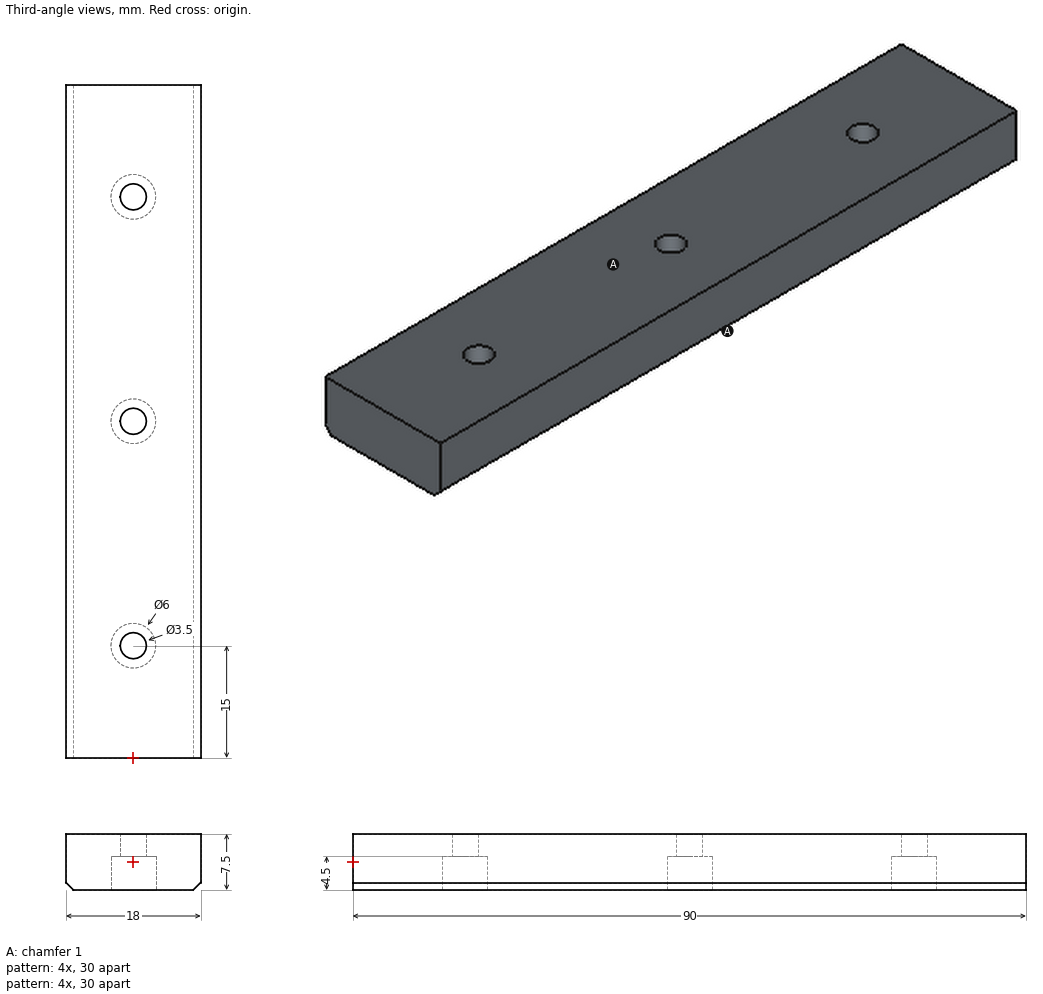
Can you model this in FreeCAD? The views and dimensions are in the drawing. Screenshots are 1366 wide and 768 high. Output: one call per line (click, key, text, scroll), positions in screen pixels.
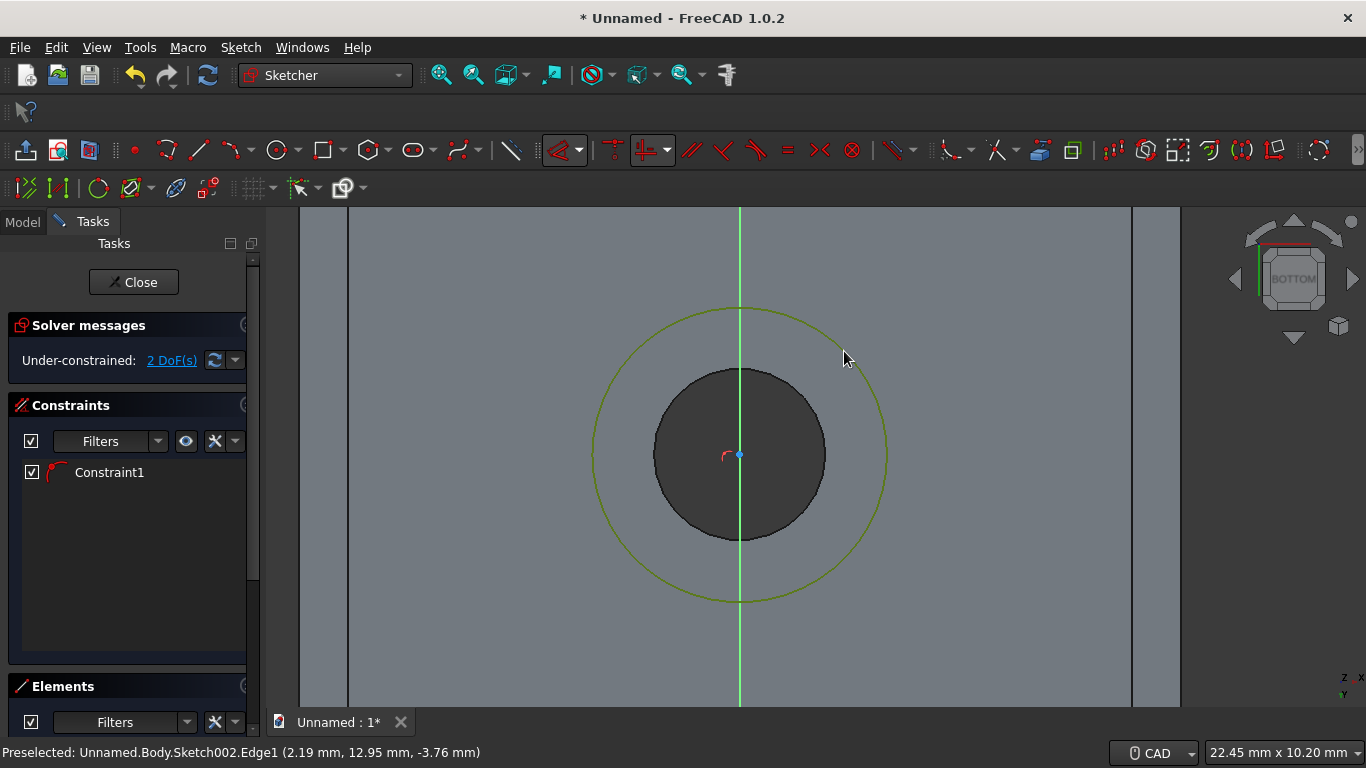
click(582, 150)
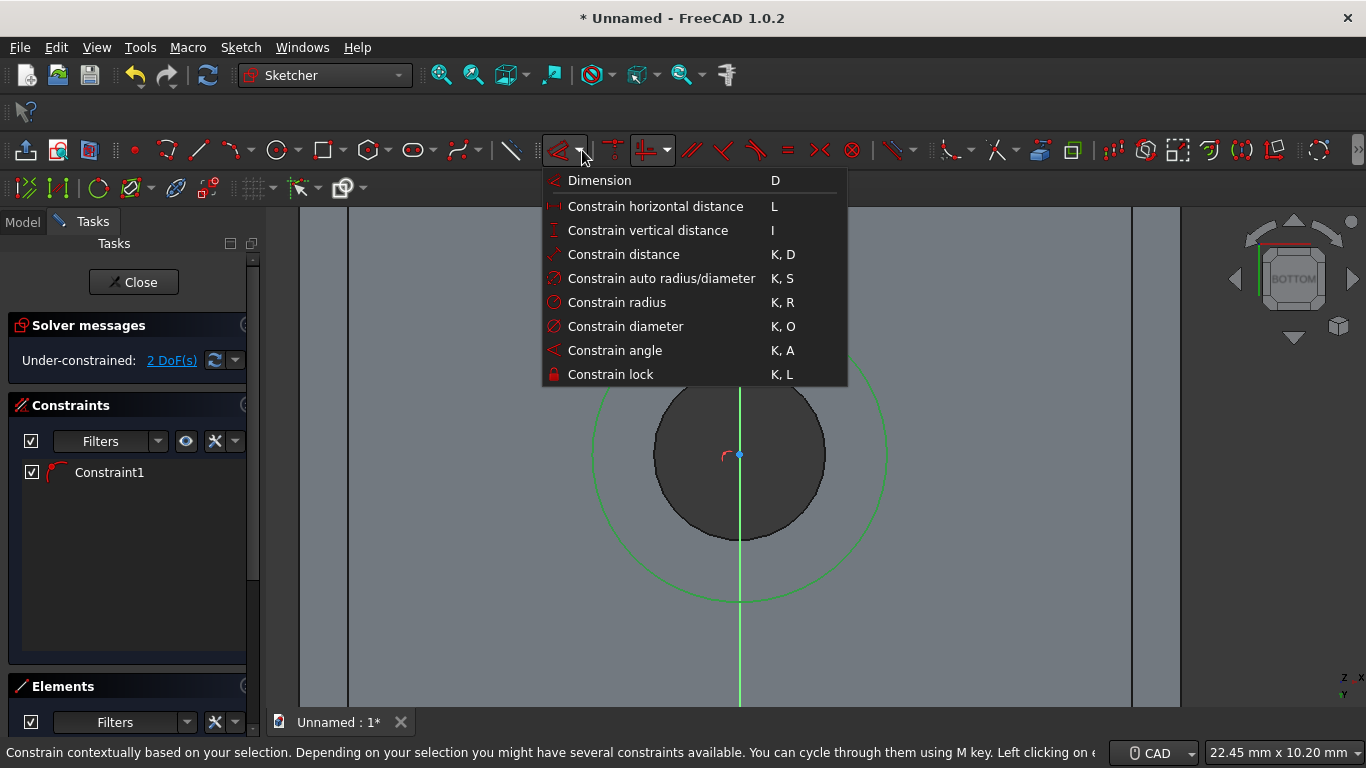
click(695, 326)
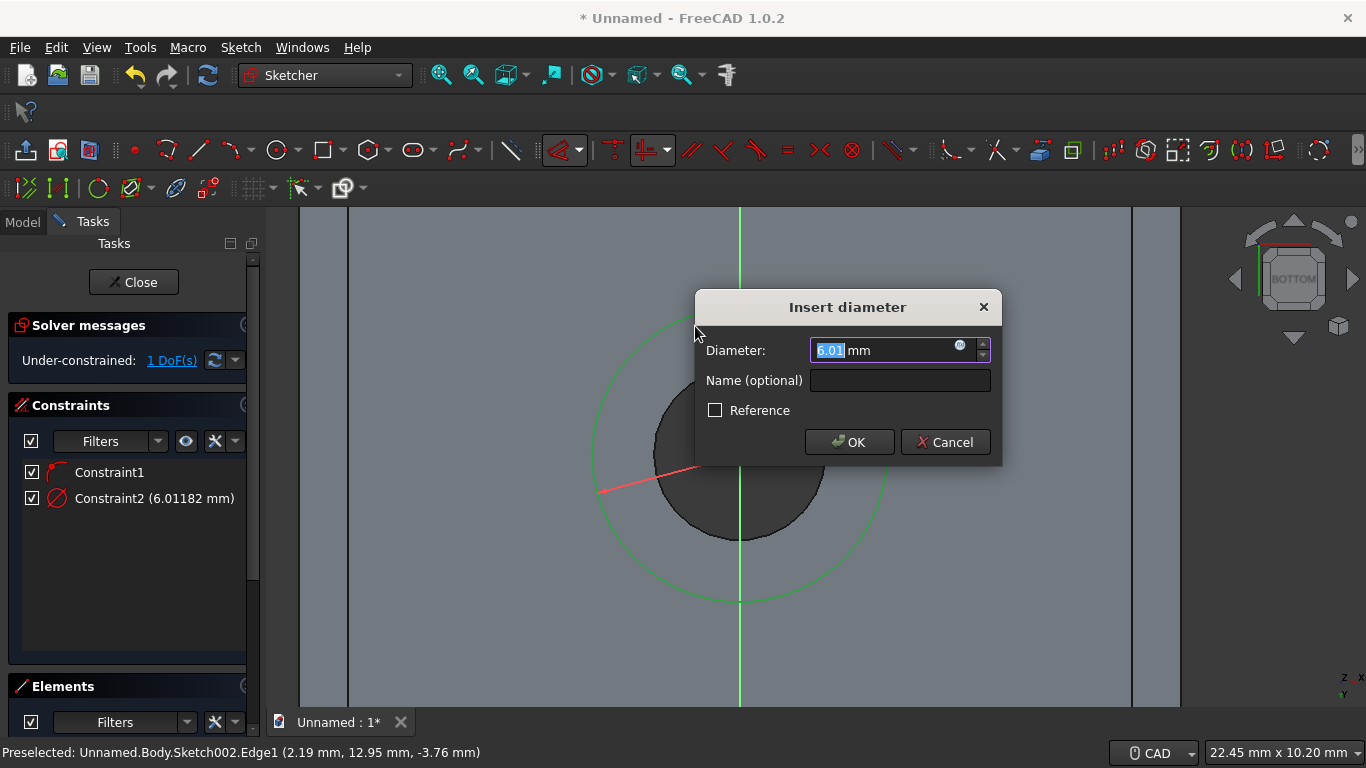
text(6)
key(Return)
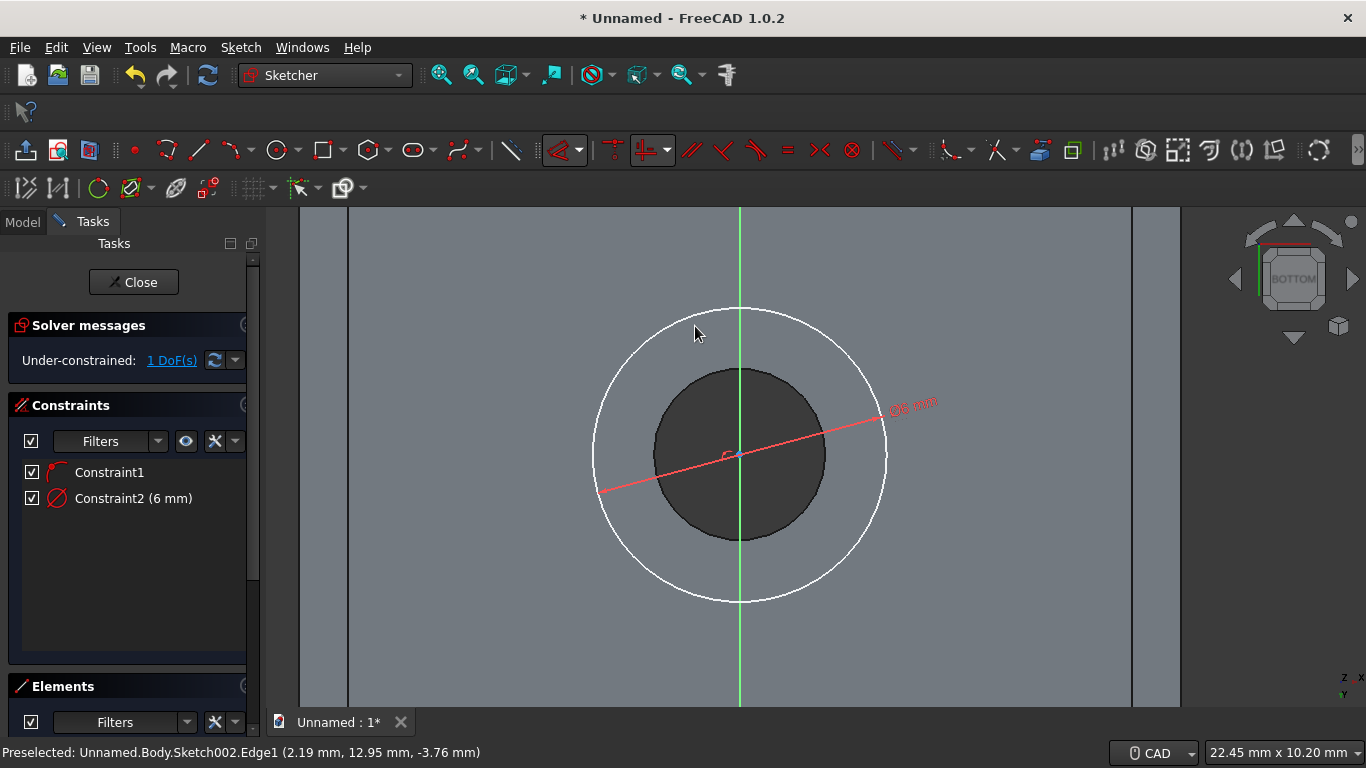
click(740, 455)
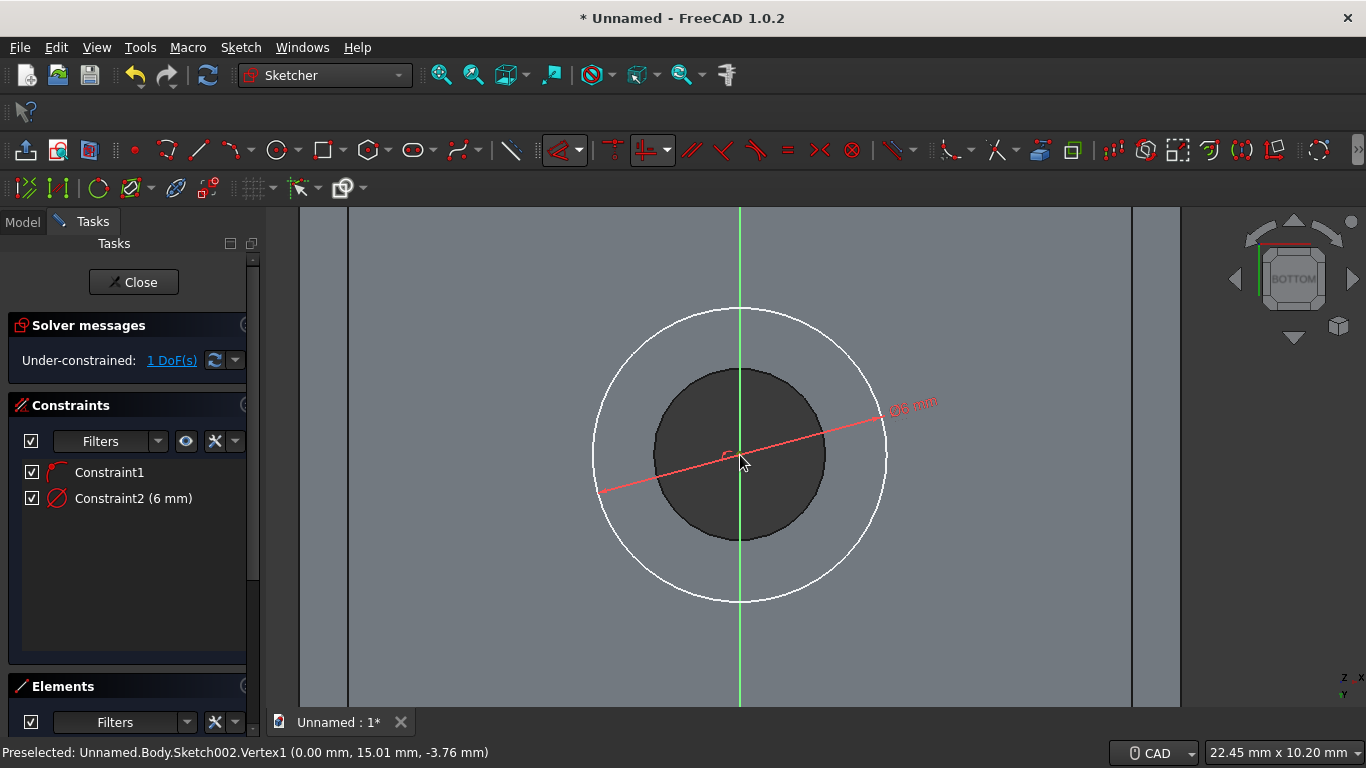
key(i)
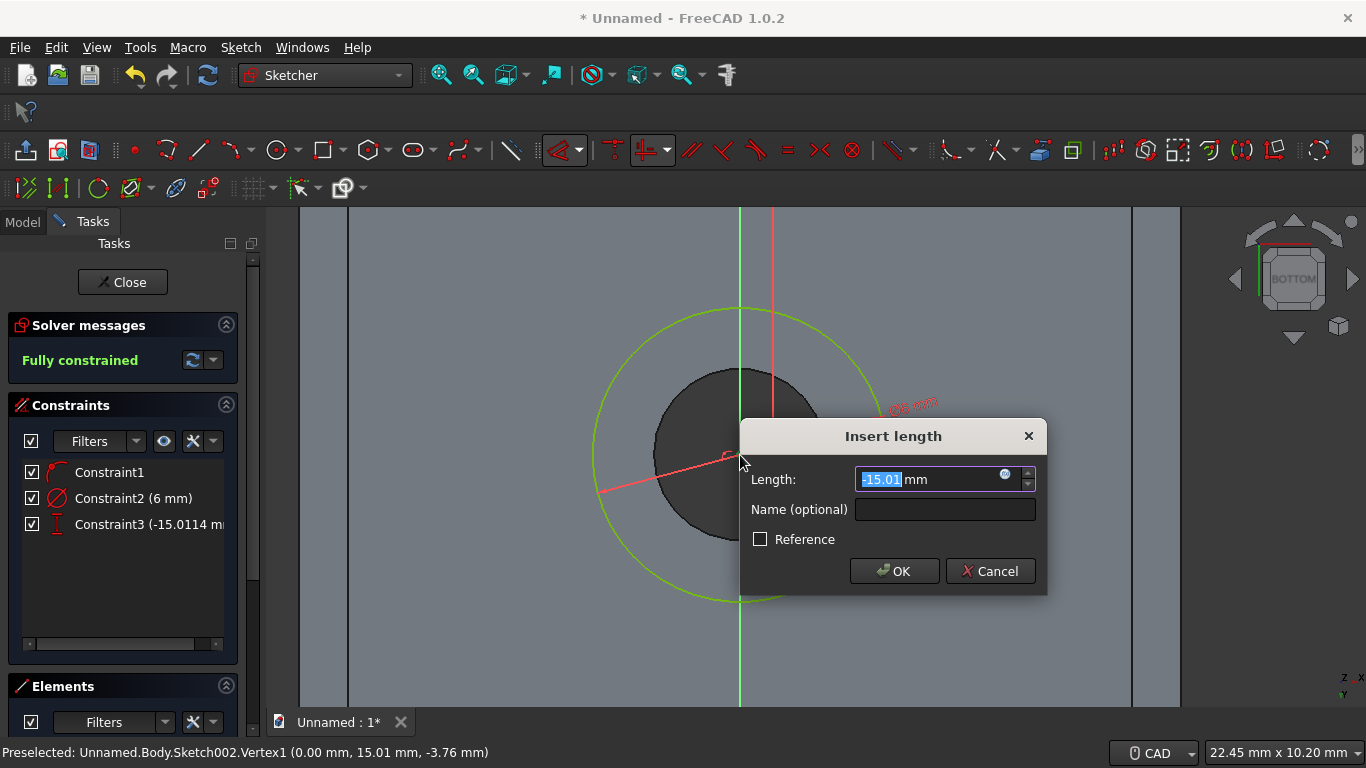
text(-15)
key(Return)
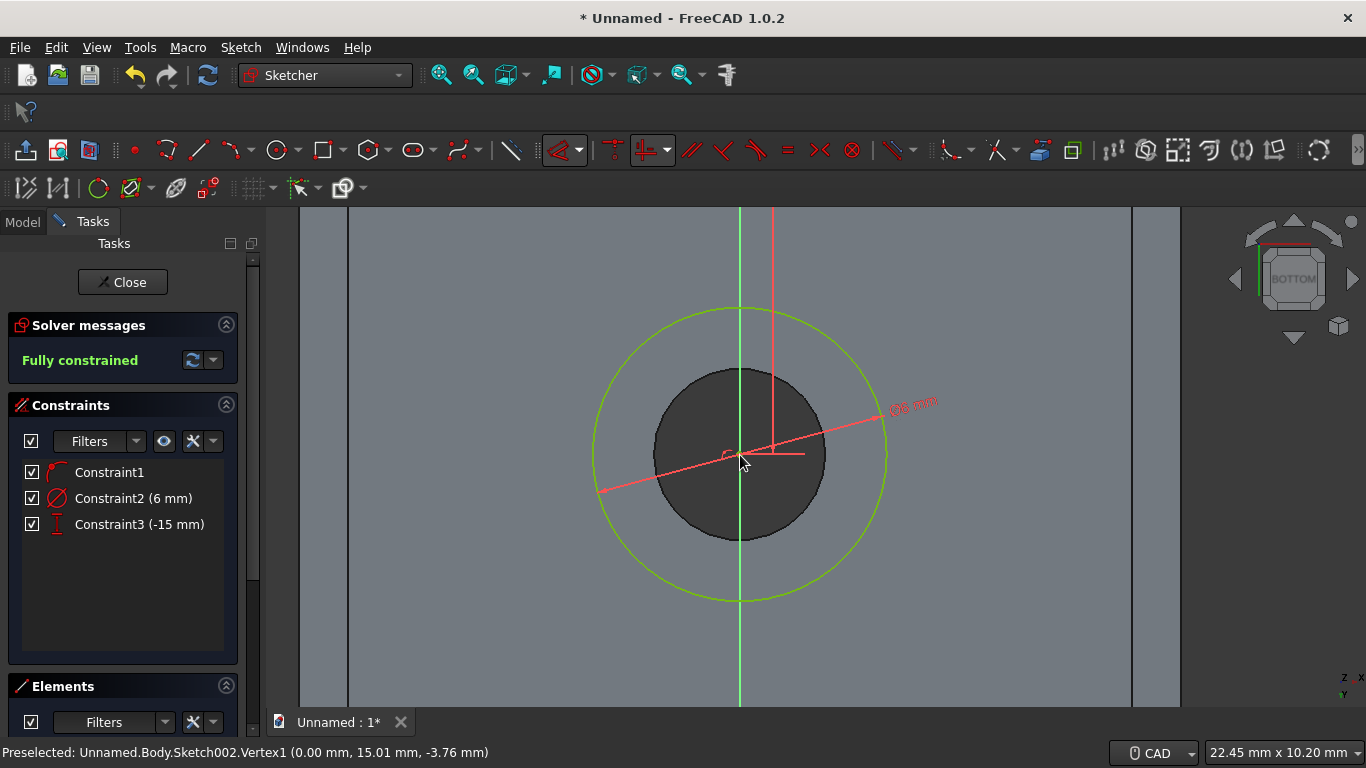
click(123, 282)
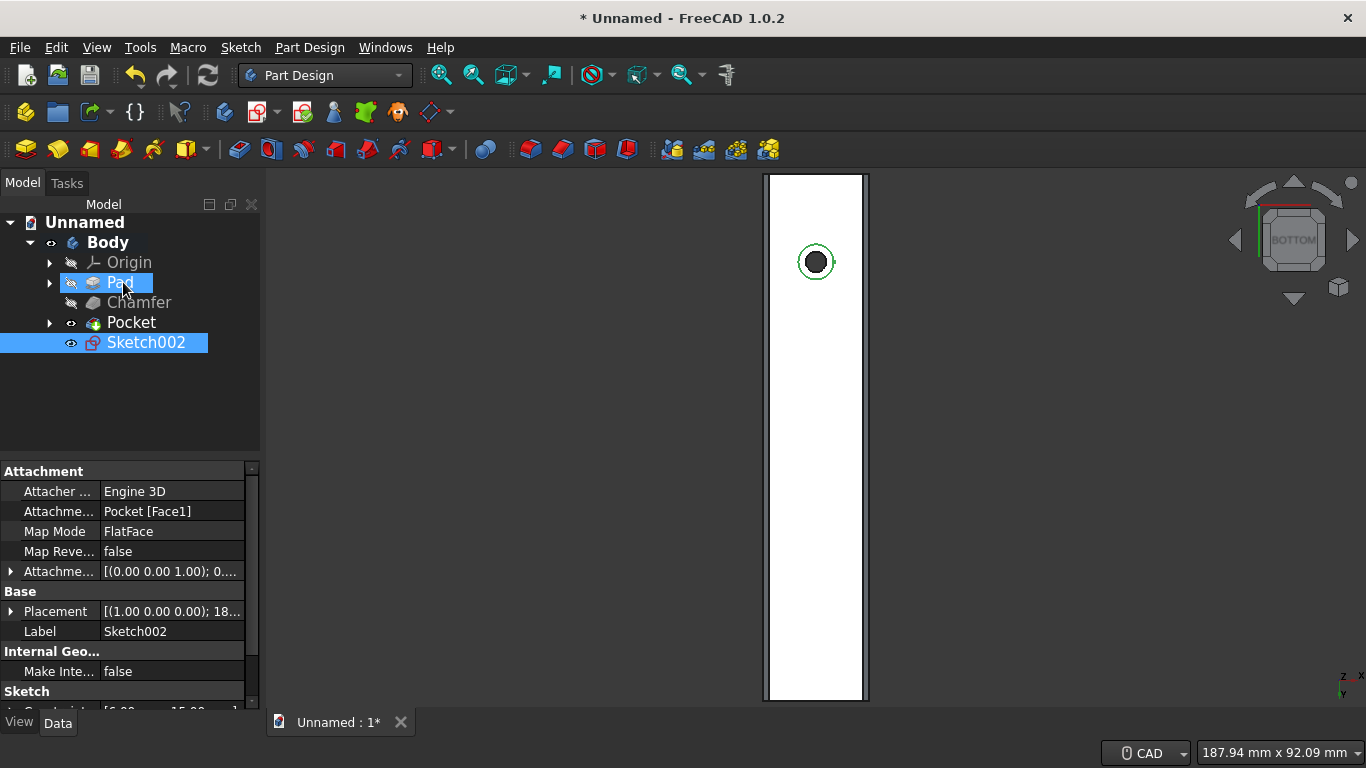
click(240, 150)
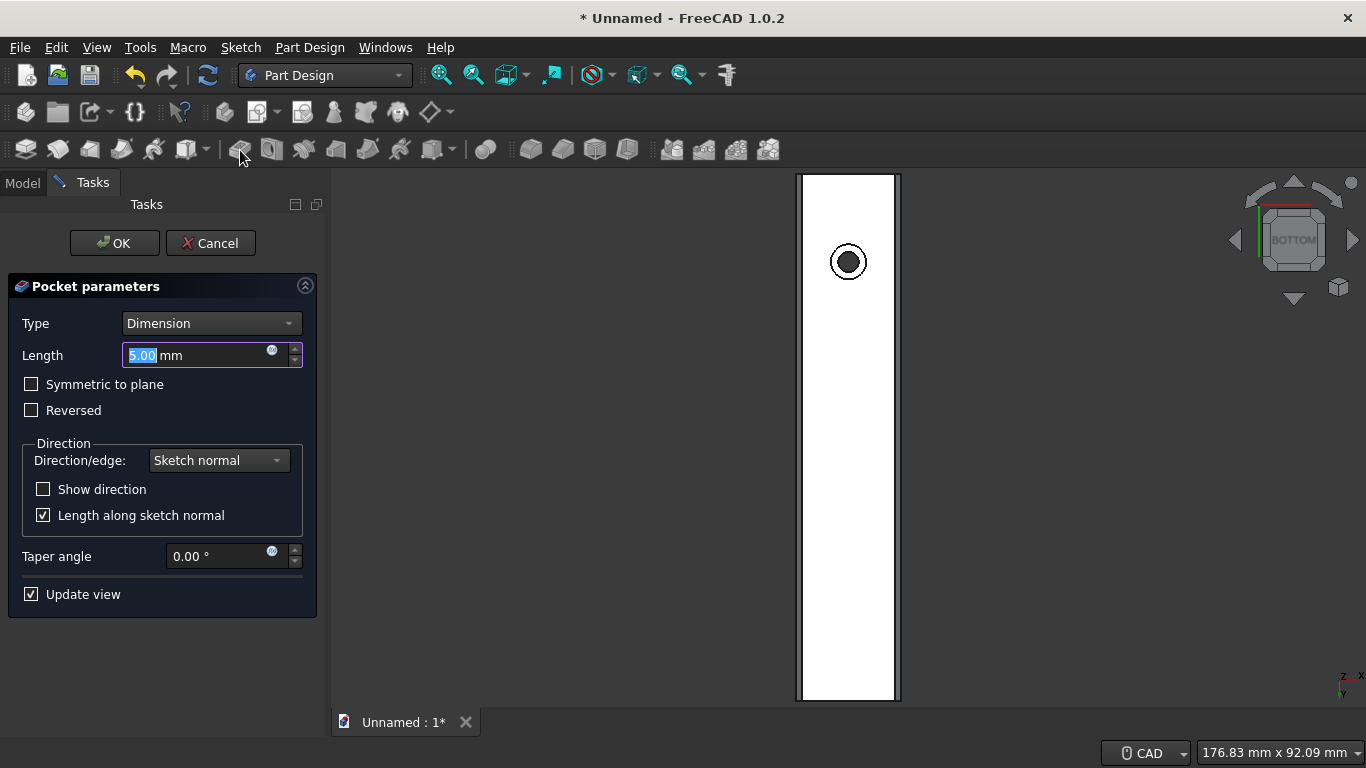
text(4.5)
key(Tab)